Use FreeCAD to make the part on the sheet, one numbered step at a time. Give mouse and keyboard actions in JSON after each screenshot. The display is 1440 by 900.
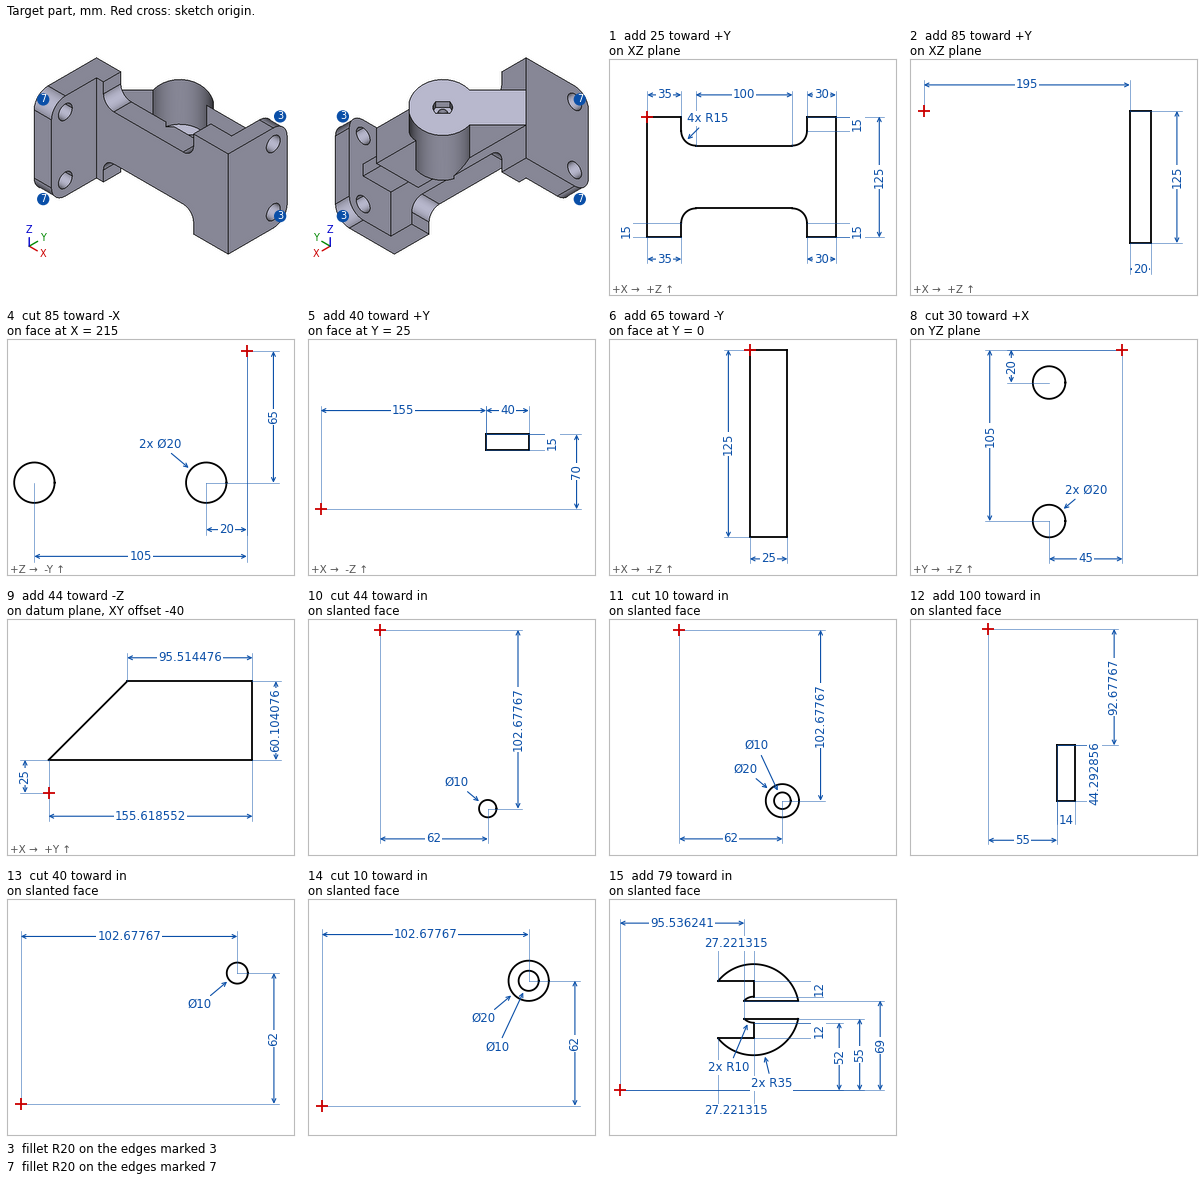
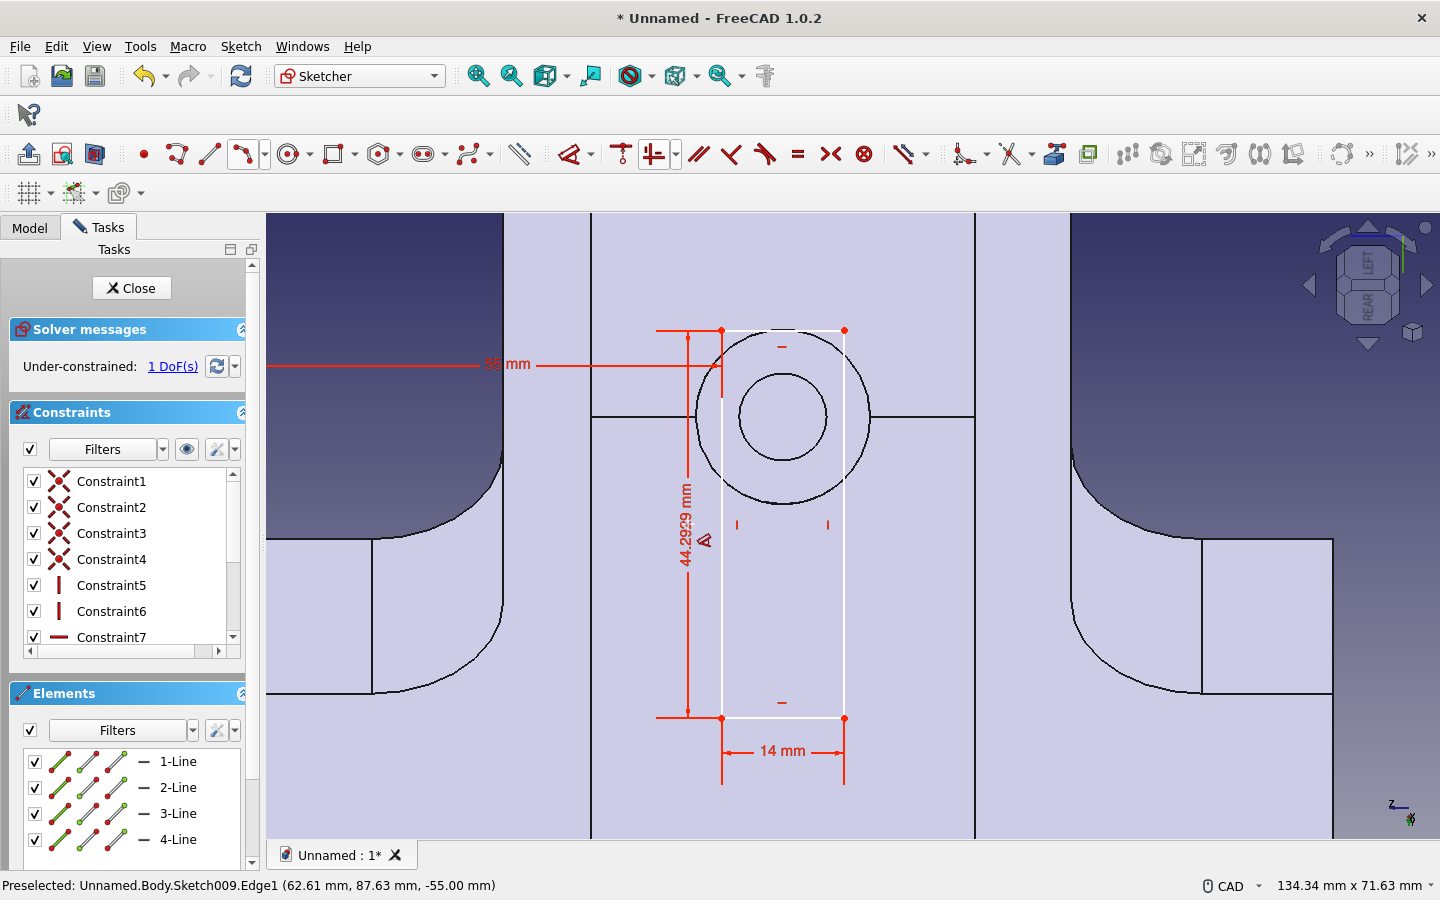
{"action": "left_click", "coordinate": [722, 331]}
{"action": "left_click", "coordinate": [756, 286]}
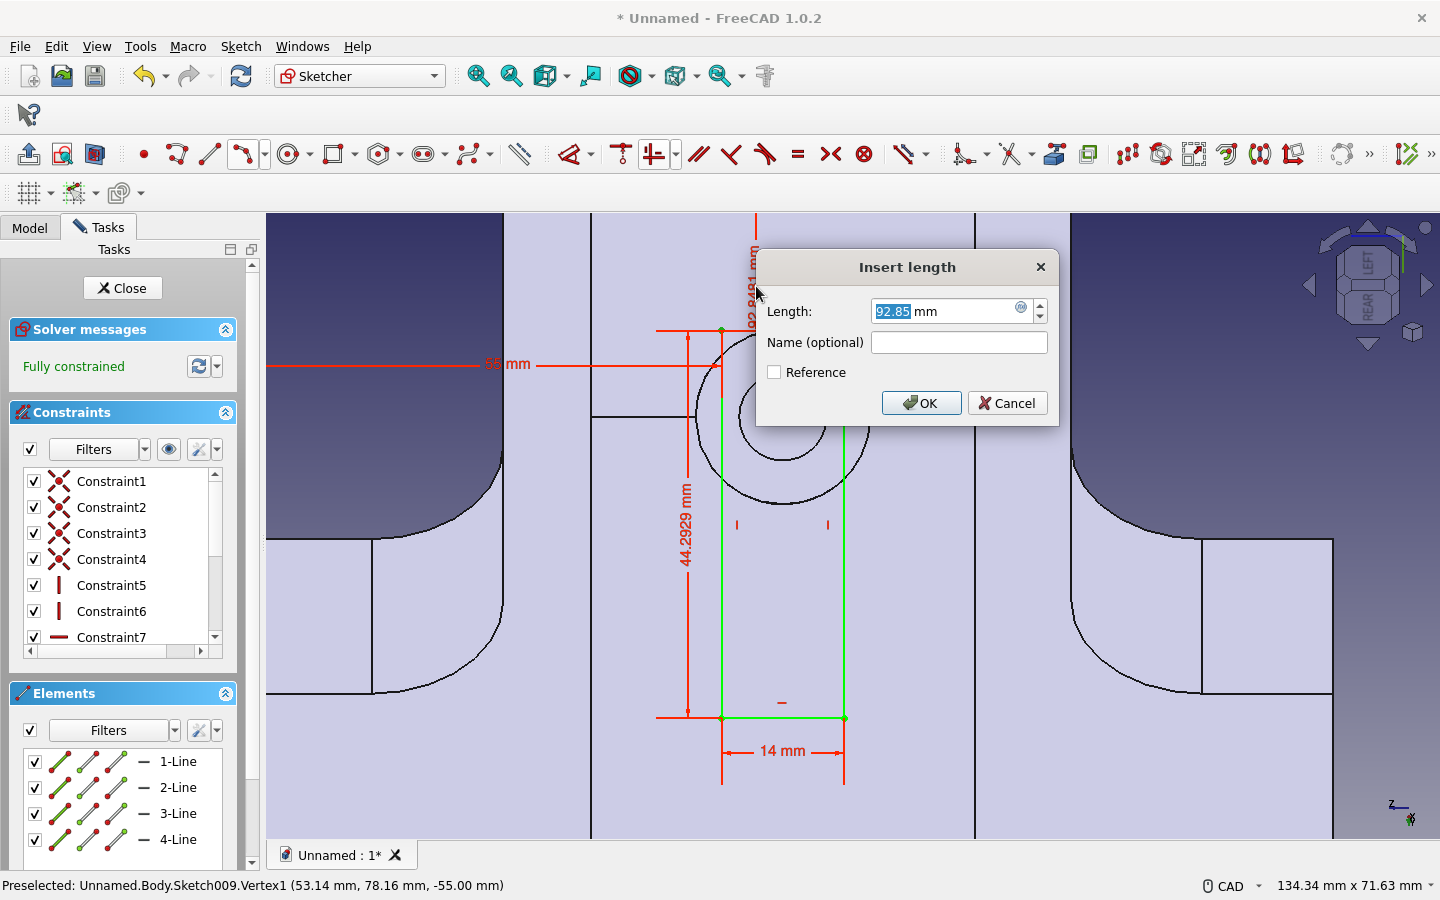
{"action": "type", "text": "92.67767"}
{"action": "key", "text": "Return"}
{"action": "key", "text": "Escape"}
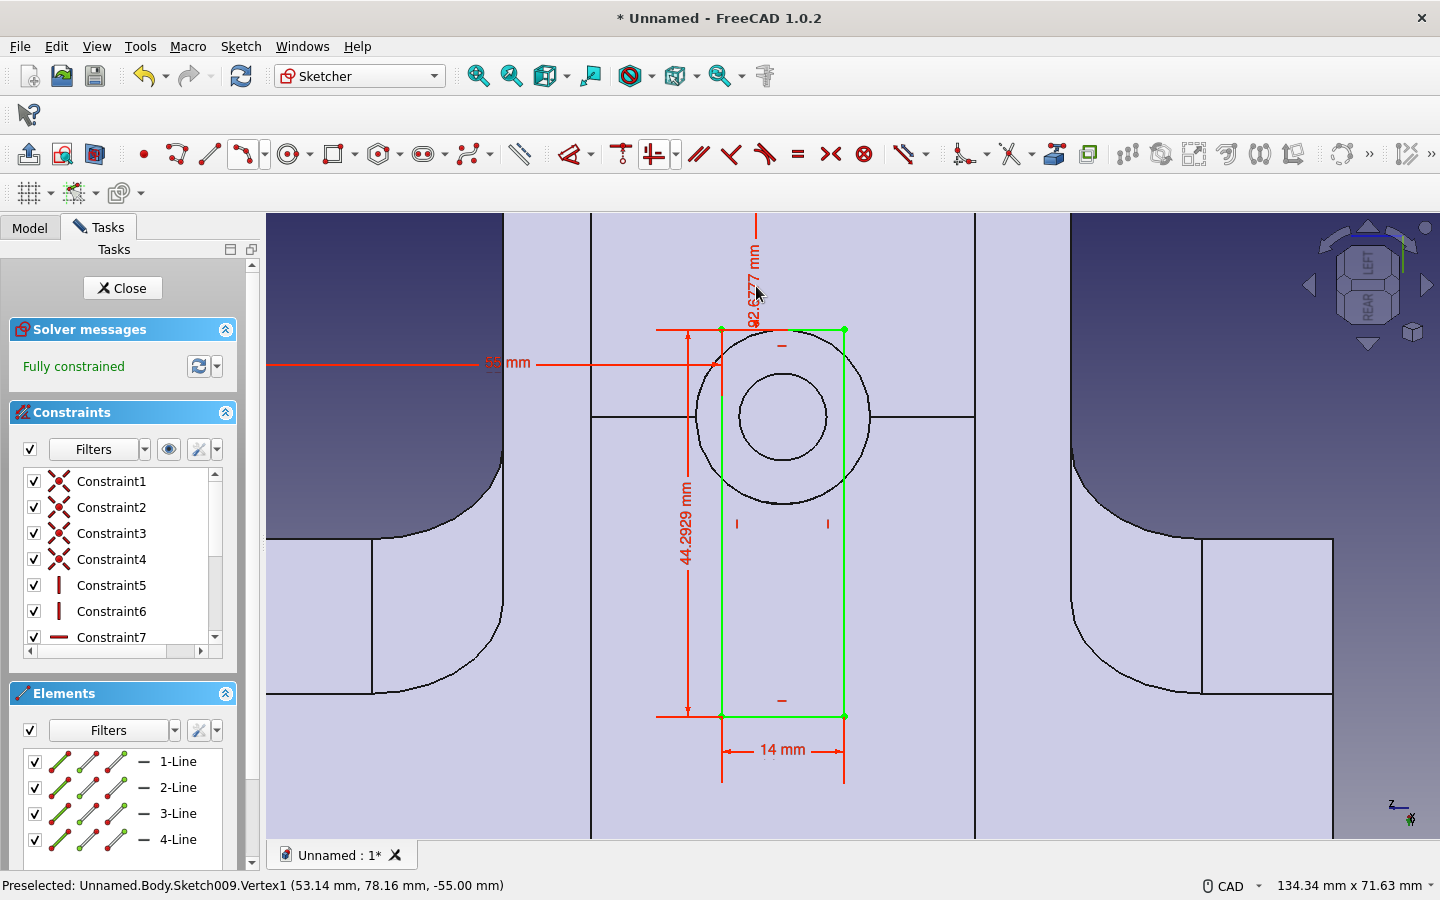
{"action": "left_click", "coordinate": [123, 288]}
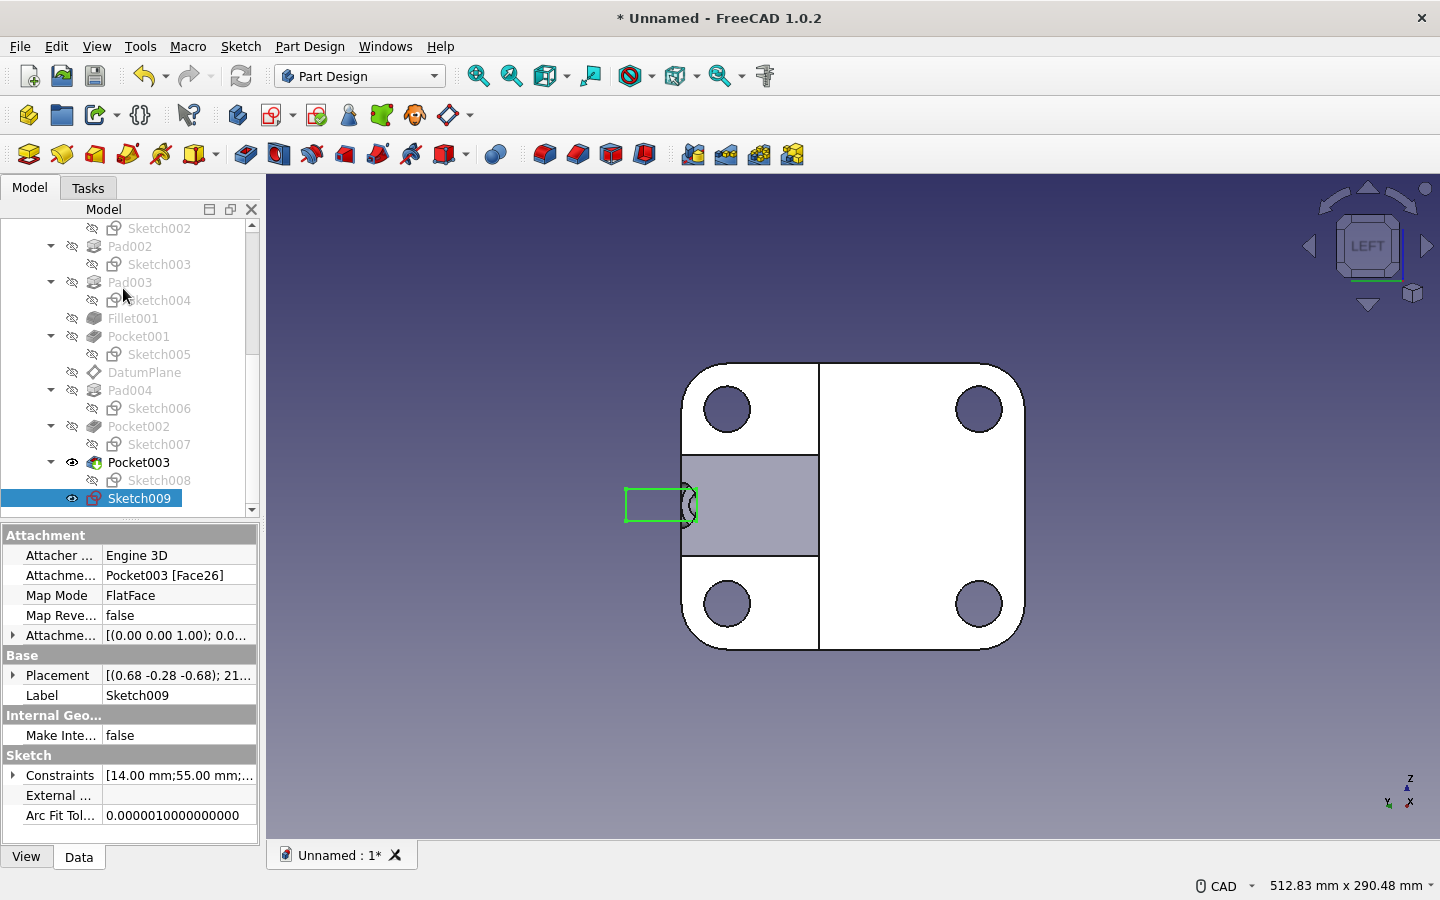
{"action": "left_click", "coordinate": [29, 154]}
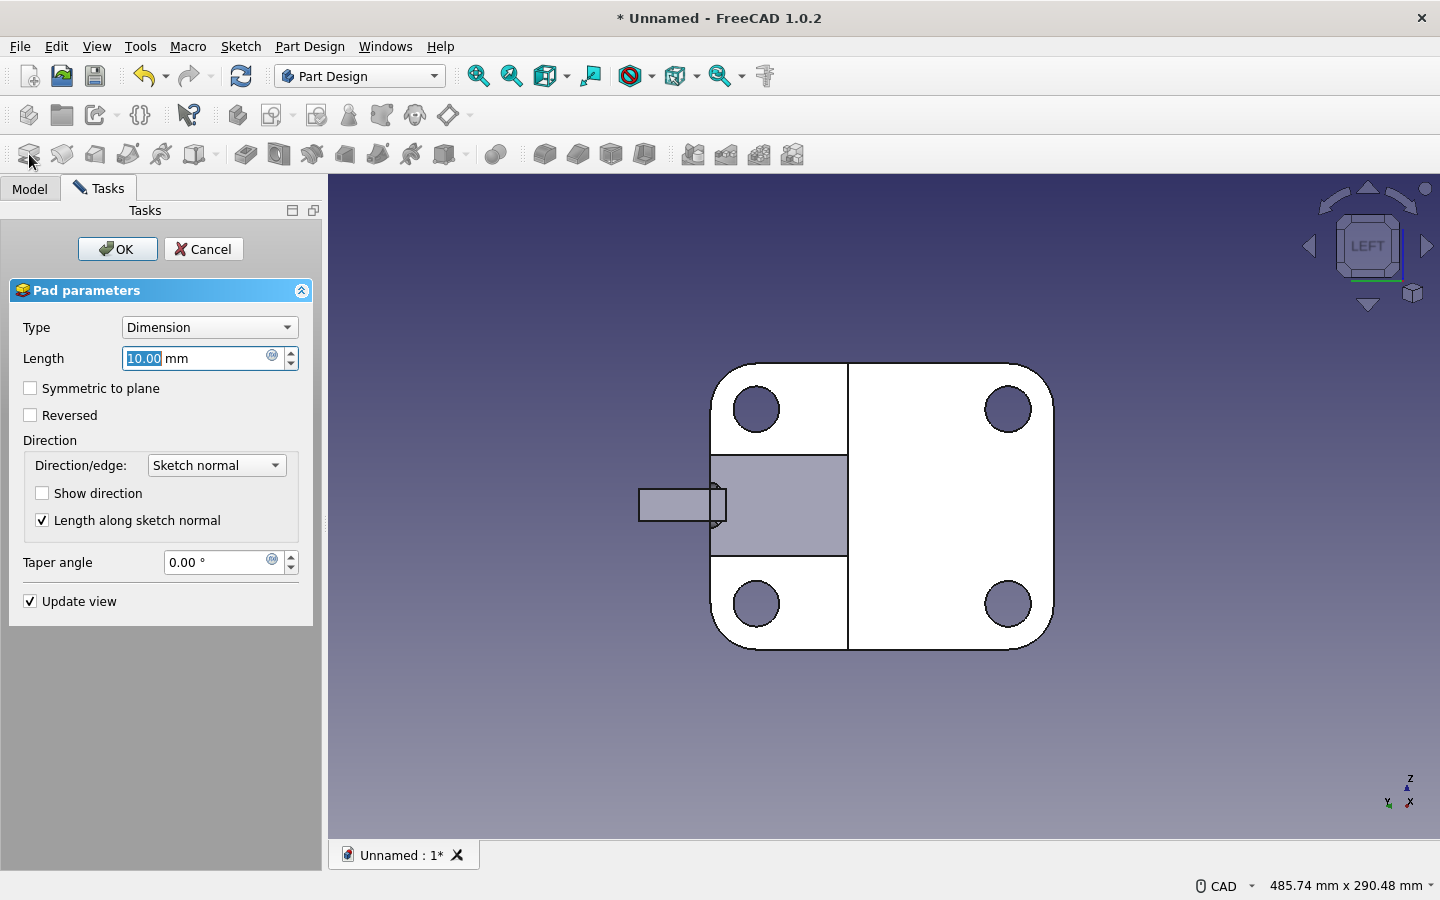
{"action": "type", "text": "100"}
{"action": "key", "text": "Tab"}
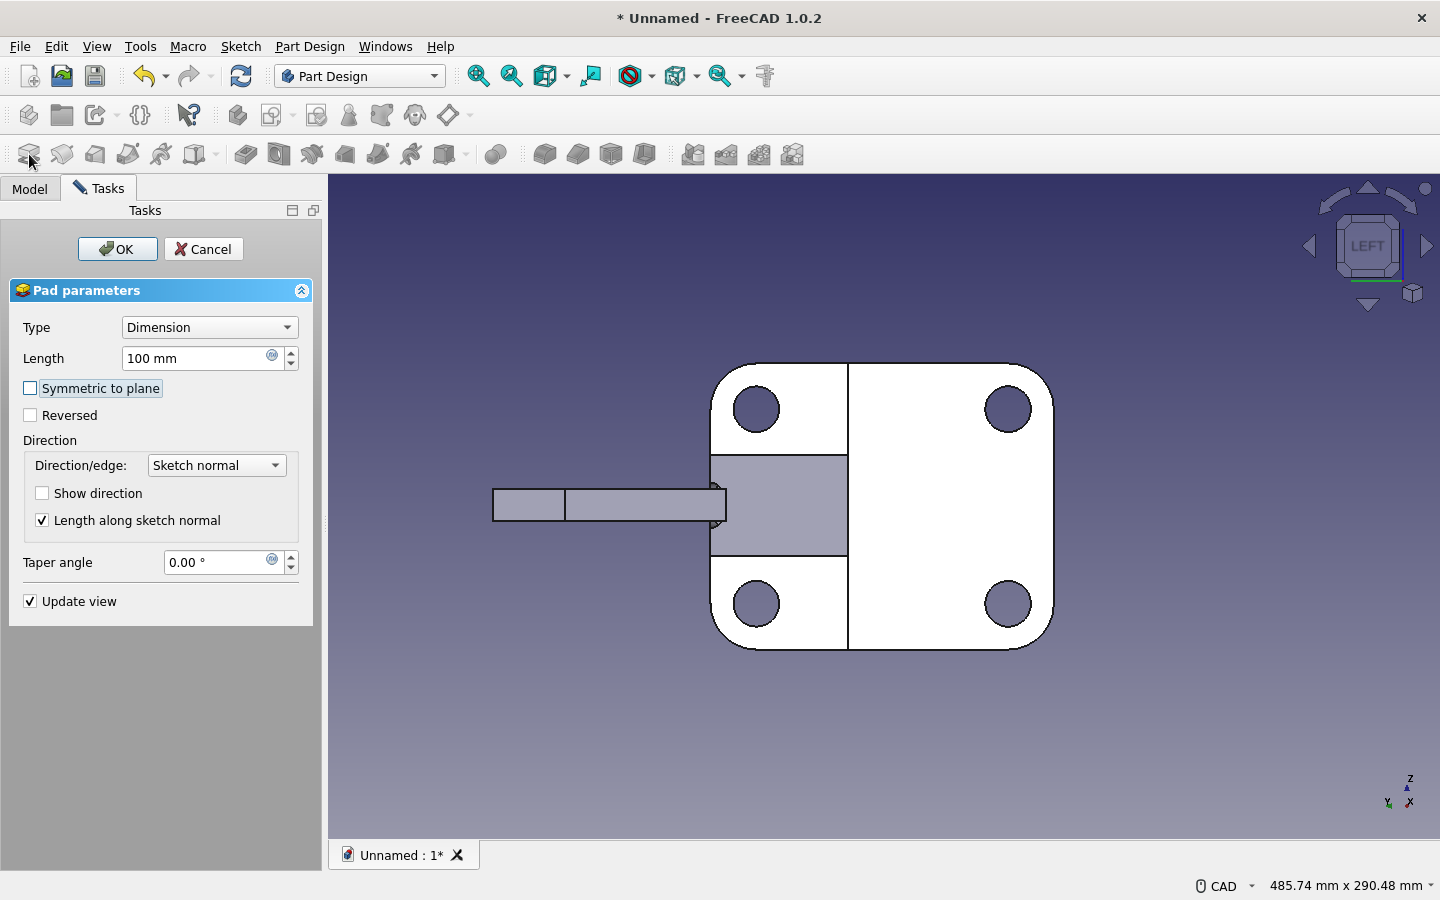
{"action": "left_click", "coordinate": [31, 415]}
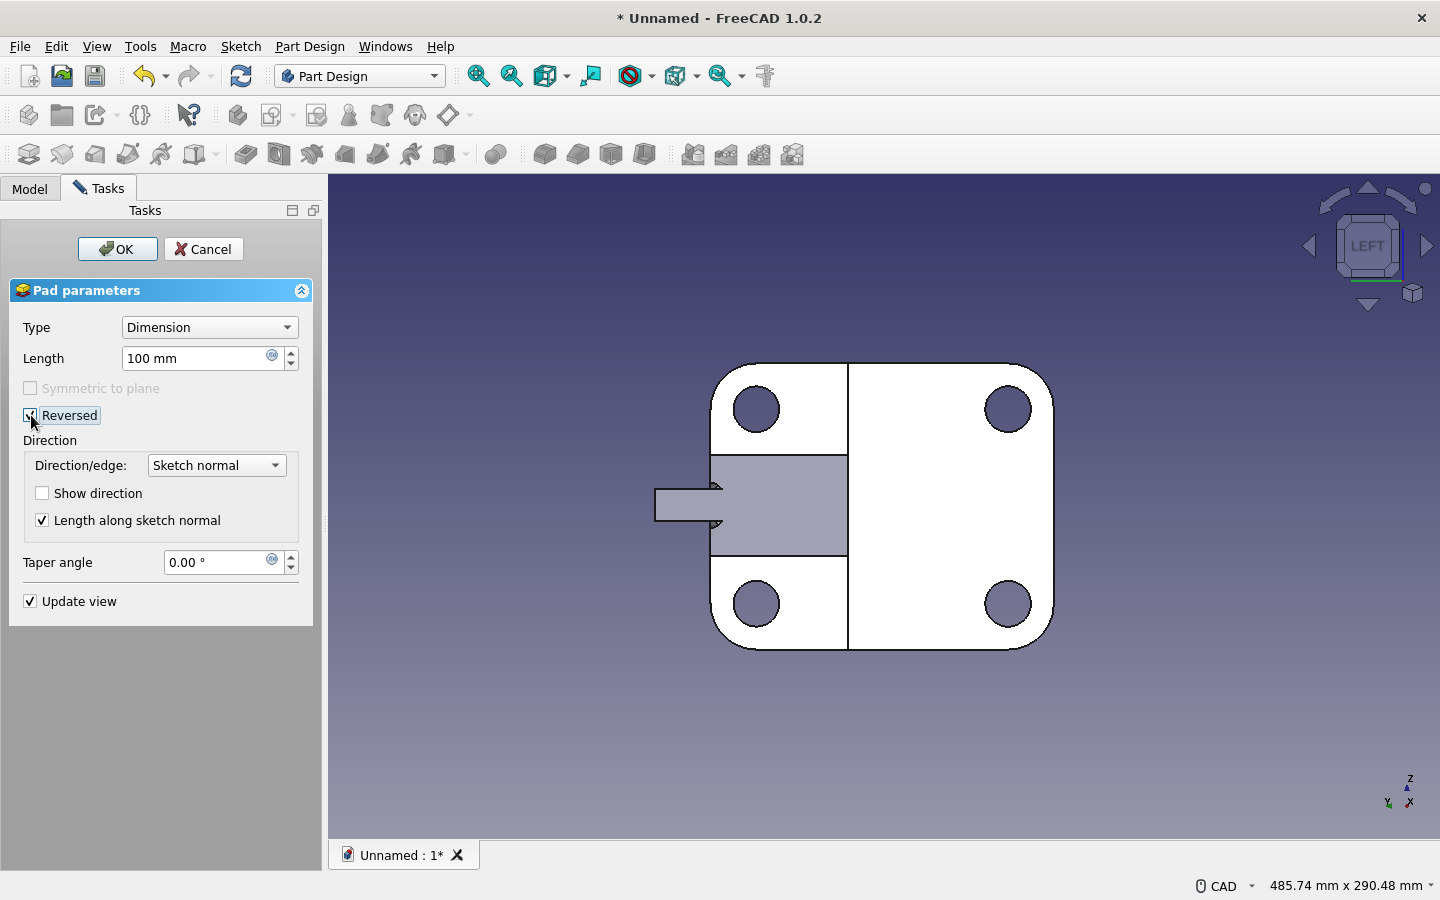
{"action": "left_click", "coordinate": [118, 249]}